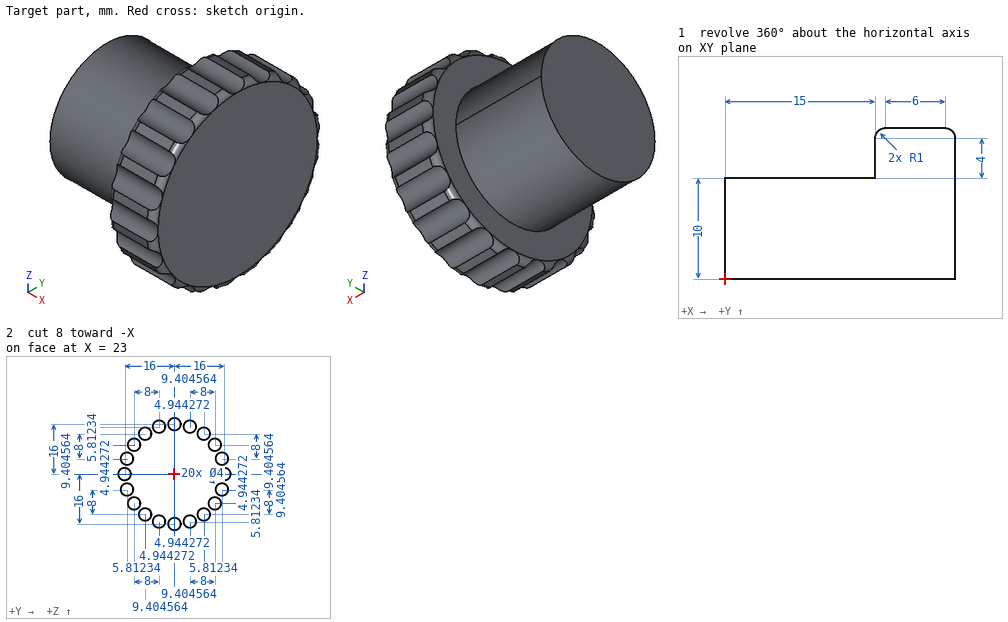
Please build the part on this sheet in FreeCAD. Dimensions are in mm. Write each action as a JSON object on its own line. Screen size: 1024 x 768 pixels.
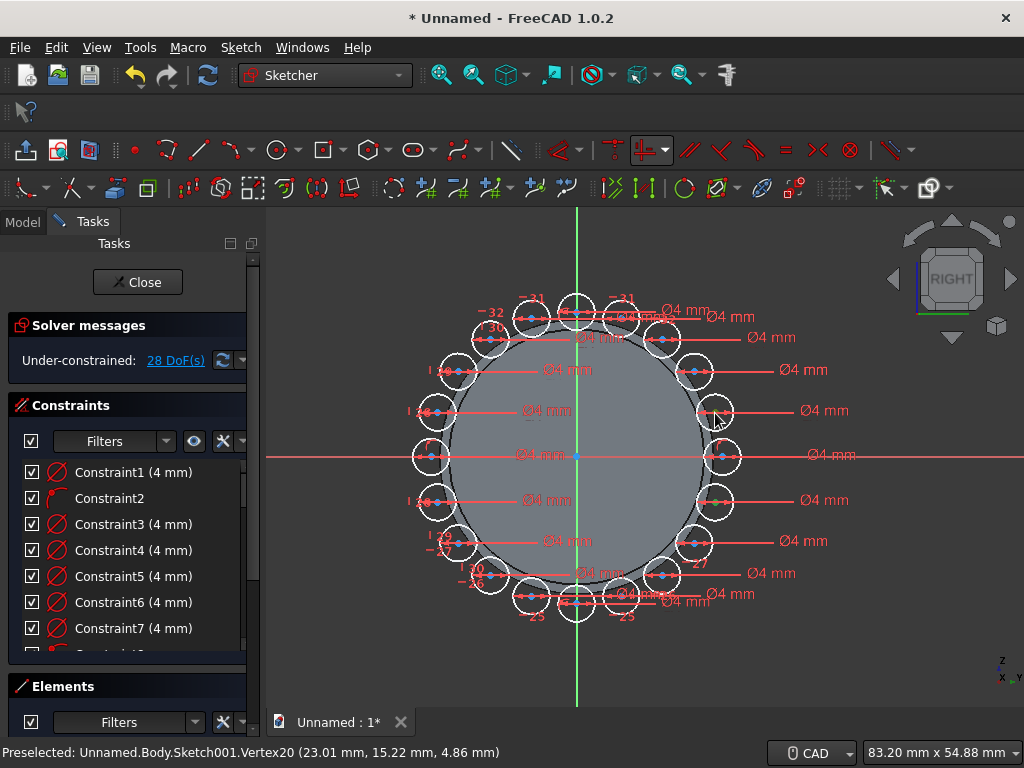
{"action": "left_click", "coordinate": [668, 150]}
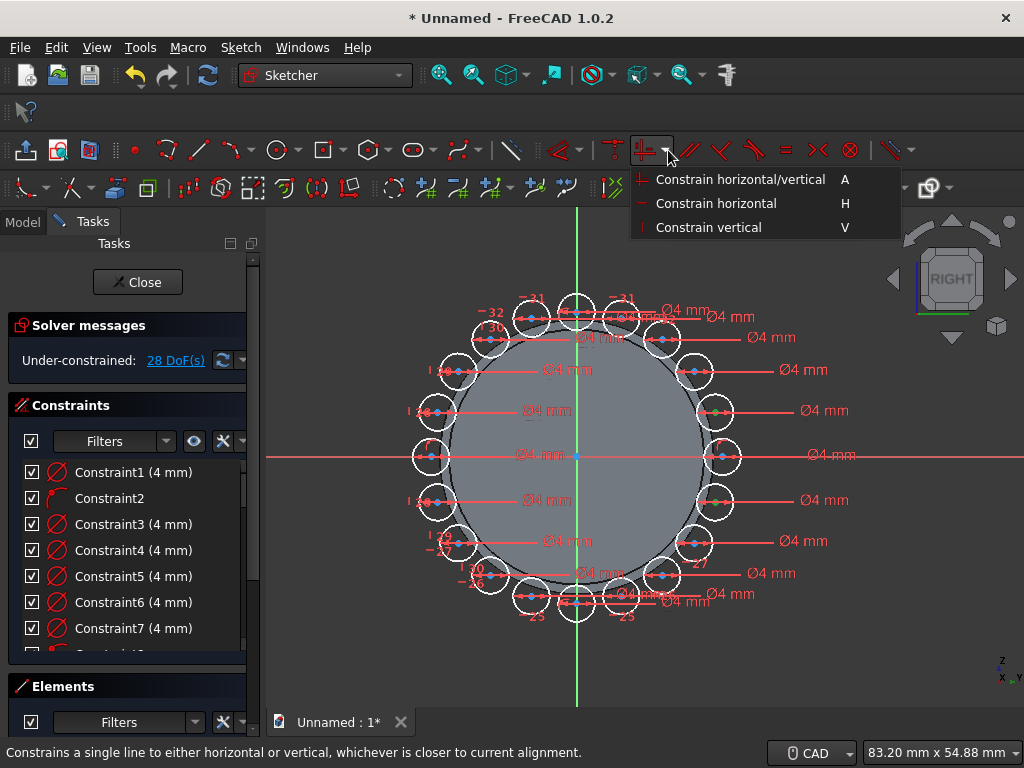
{"action": "left_click", "coordinate": [766, 227]}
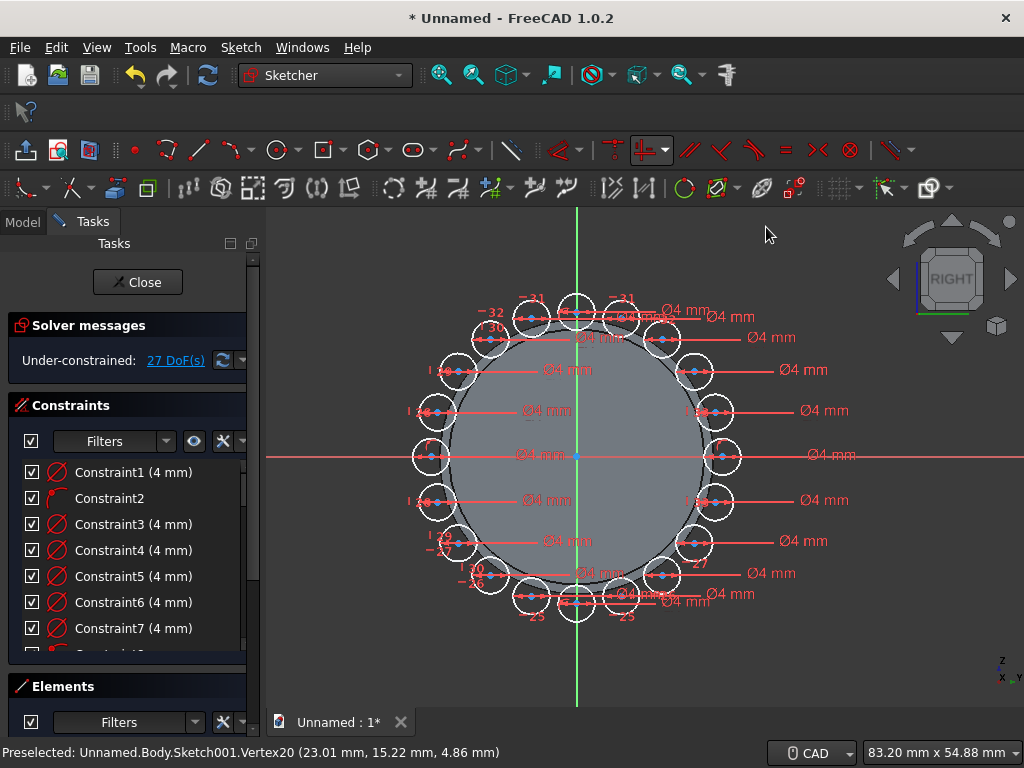
{"action": "left_click", "coordinate": [558, 150]}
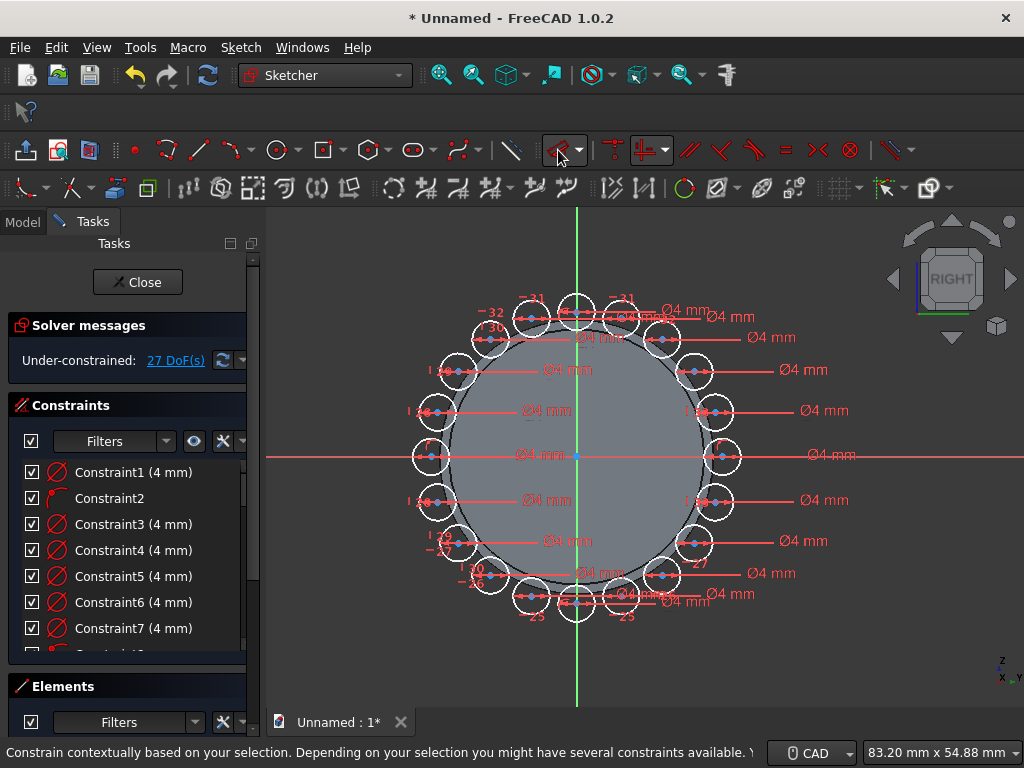
{"action": "left_click", "coordinate": [723, 457]}
{"action": "left_click", "coordinate": [650, 491]}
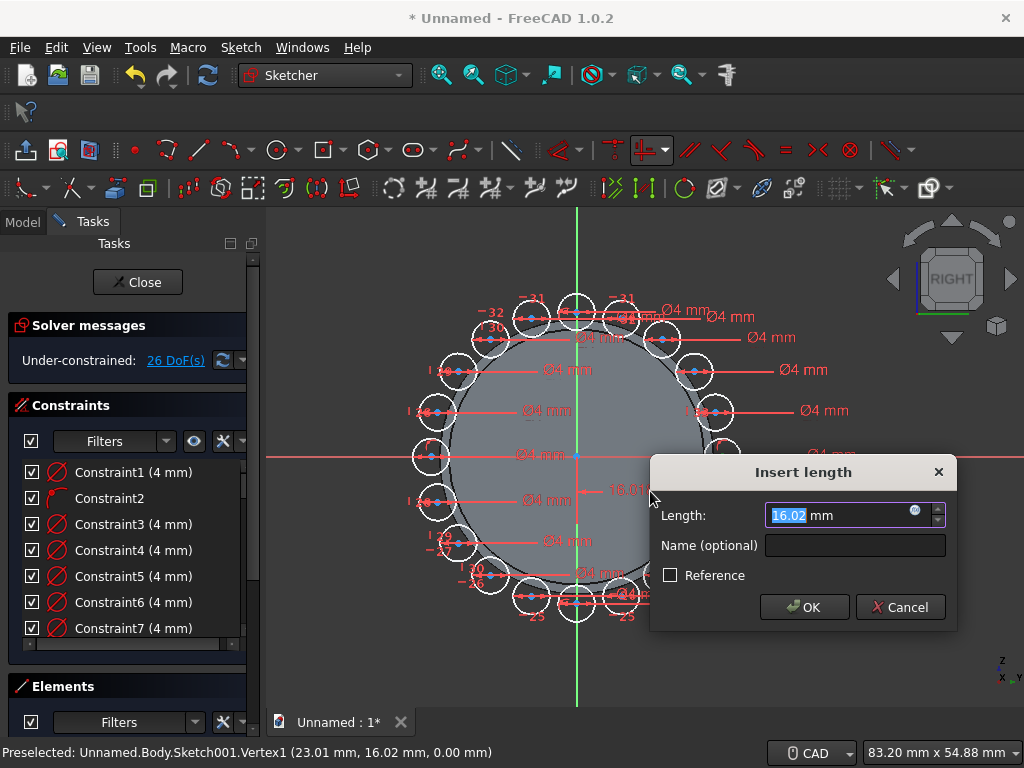
{"action": "type", "text": "16"}
{"action": "key", "text": "Return"}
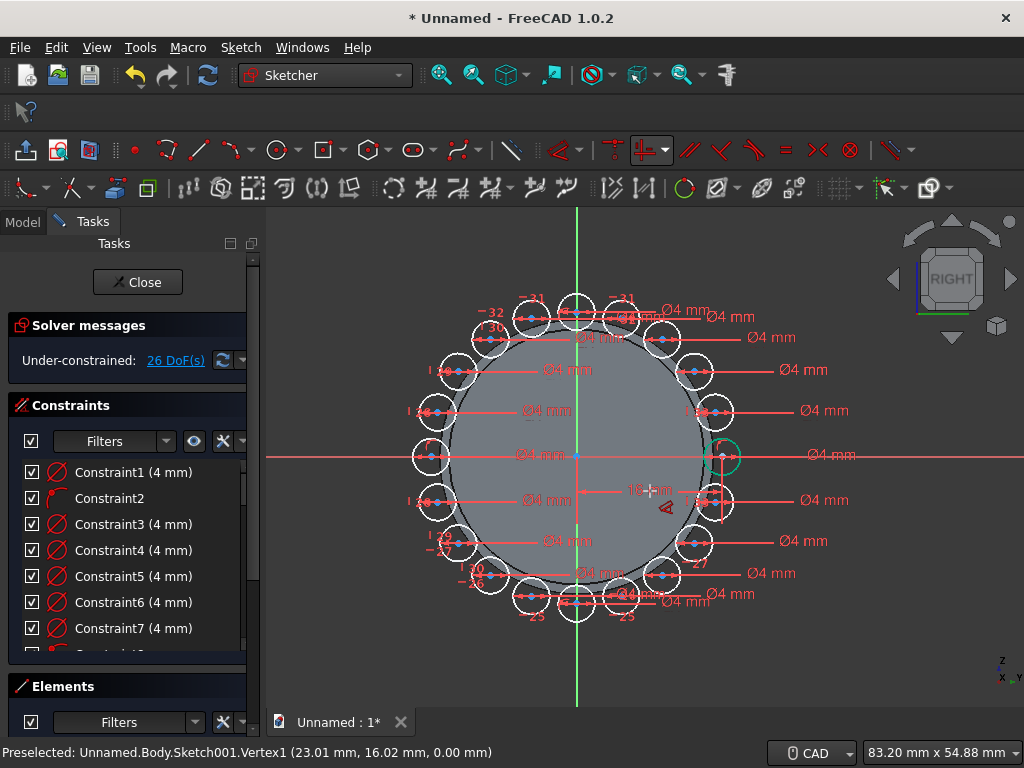
{"action": "left_click", "coordinate": [577, 604]}
{"action": "left_click", "coordinate": [611, 530]}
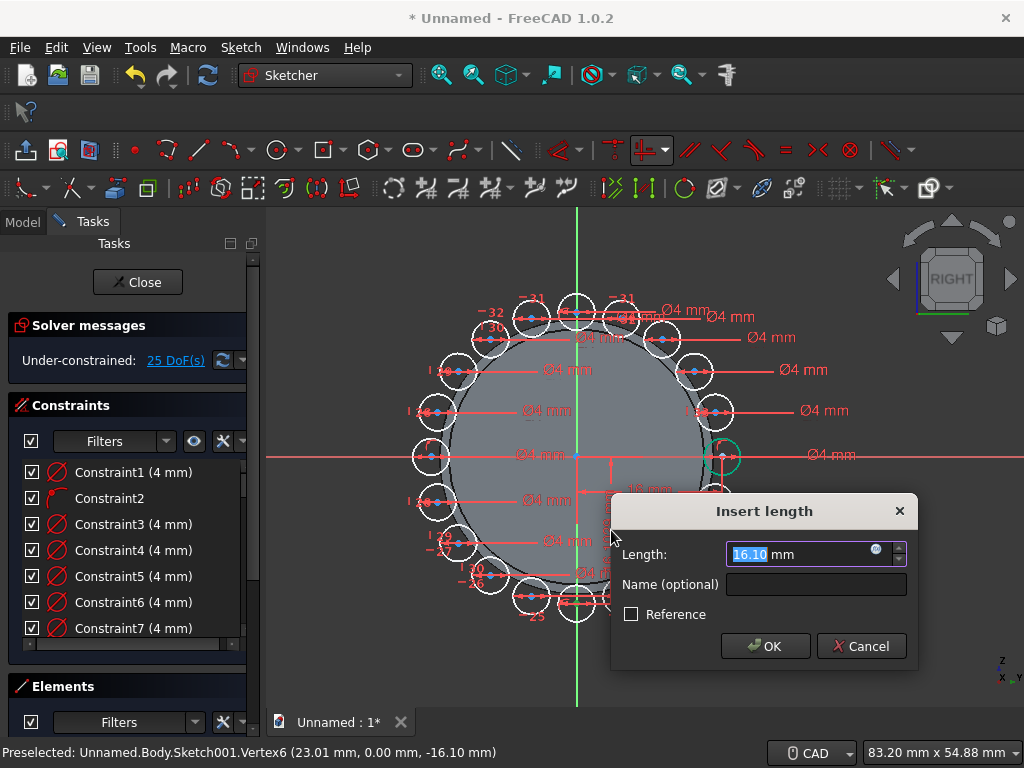
{"action": "type", "text": "16"}
{"action": "key", "text": "Return"}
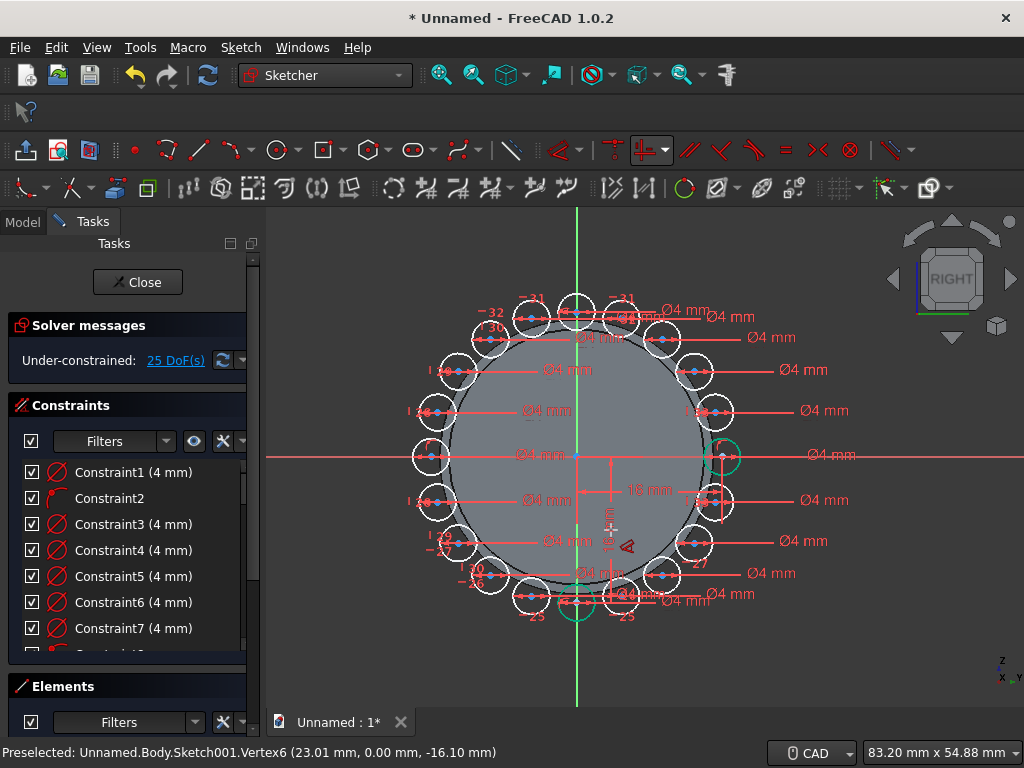
{"action": "left_click", "coordinate": [431, 457]}
{"action": "left_click", "coordinate": [504, 491]}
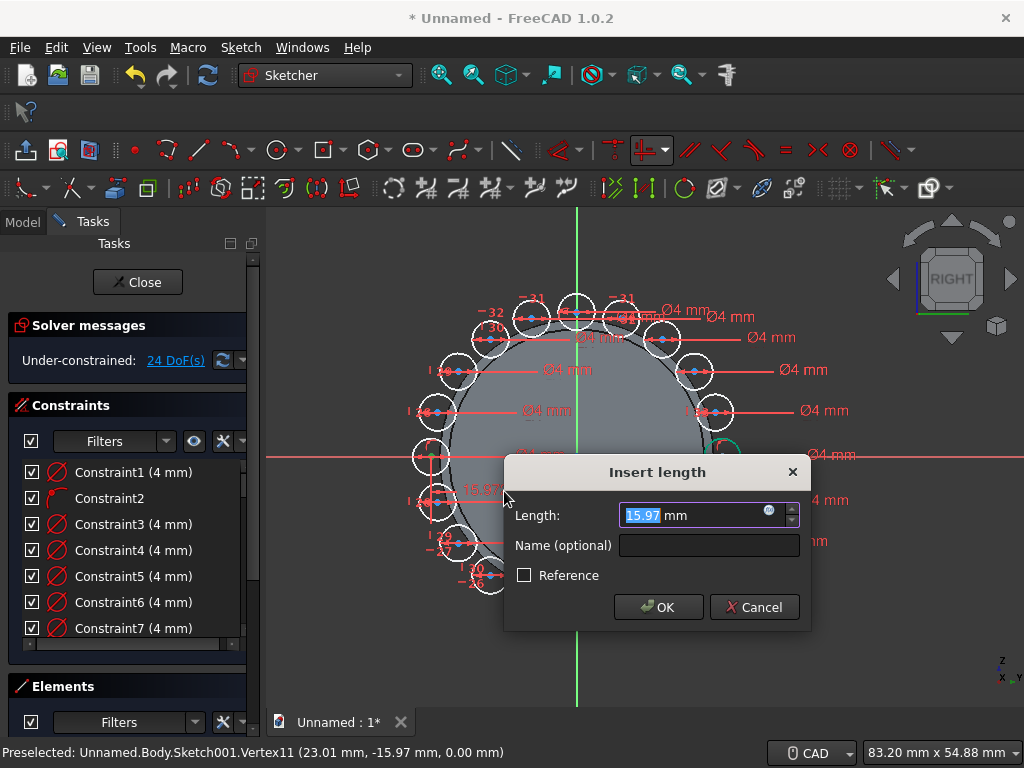
{"action": "type", "text": "16"}
{"action": "key", "text": "Return"}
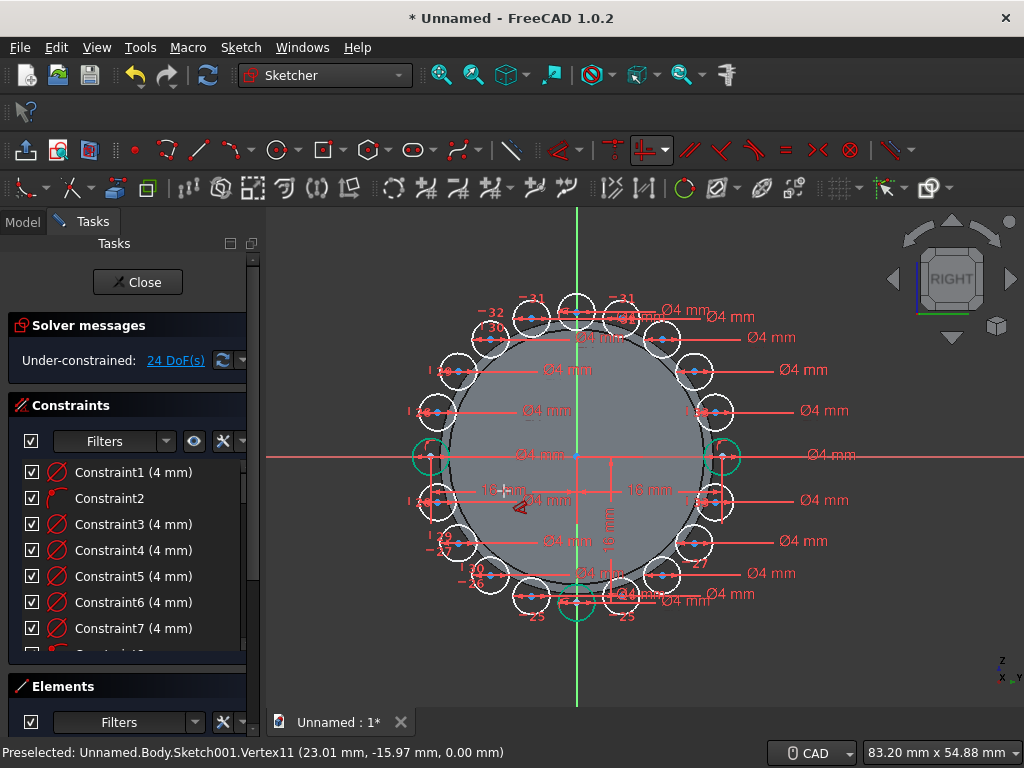
{"action": "left_click", "coordinate": [577, 312]}
{"action": "left_click", "coordinate": [611, 384]}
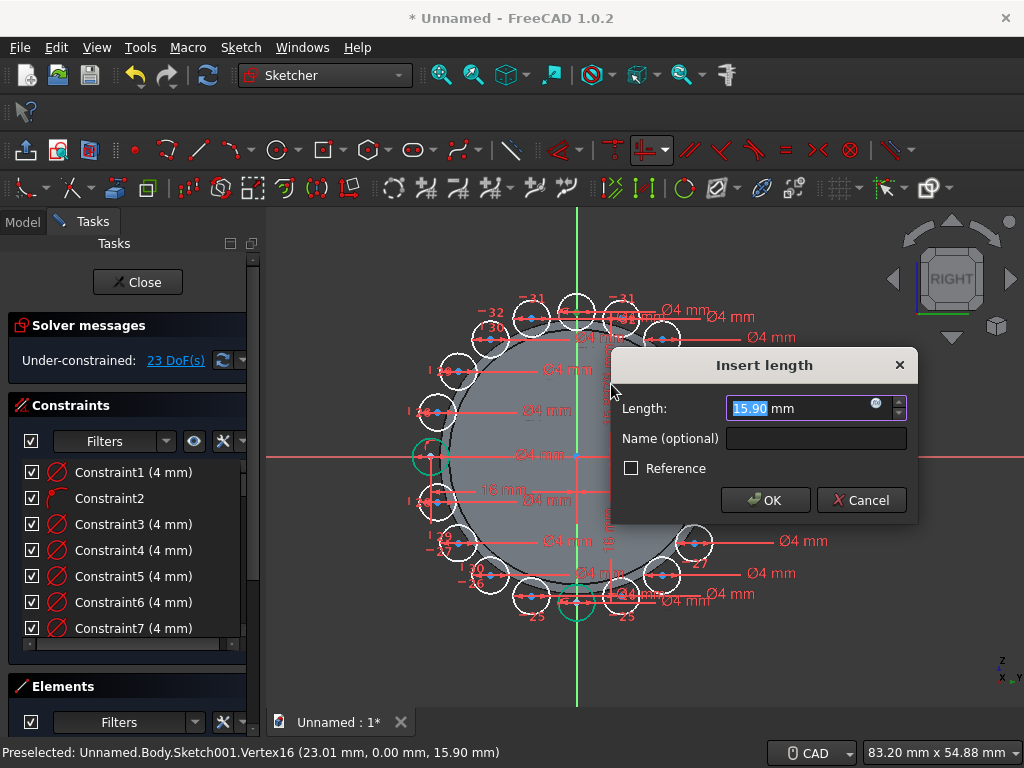
{"action": "type", "text": "16"}
{"action": "key", "text": "Return"}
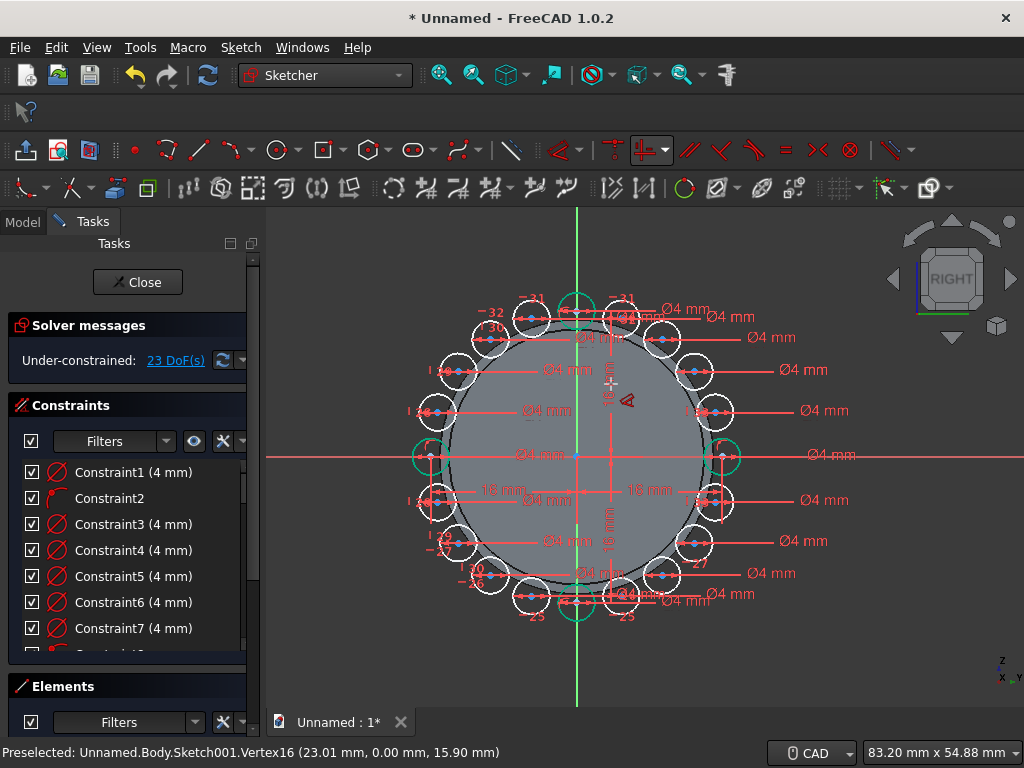
{"action": "left_click", "coordinate": [715, 502]}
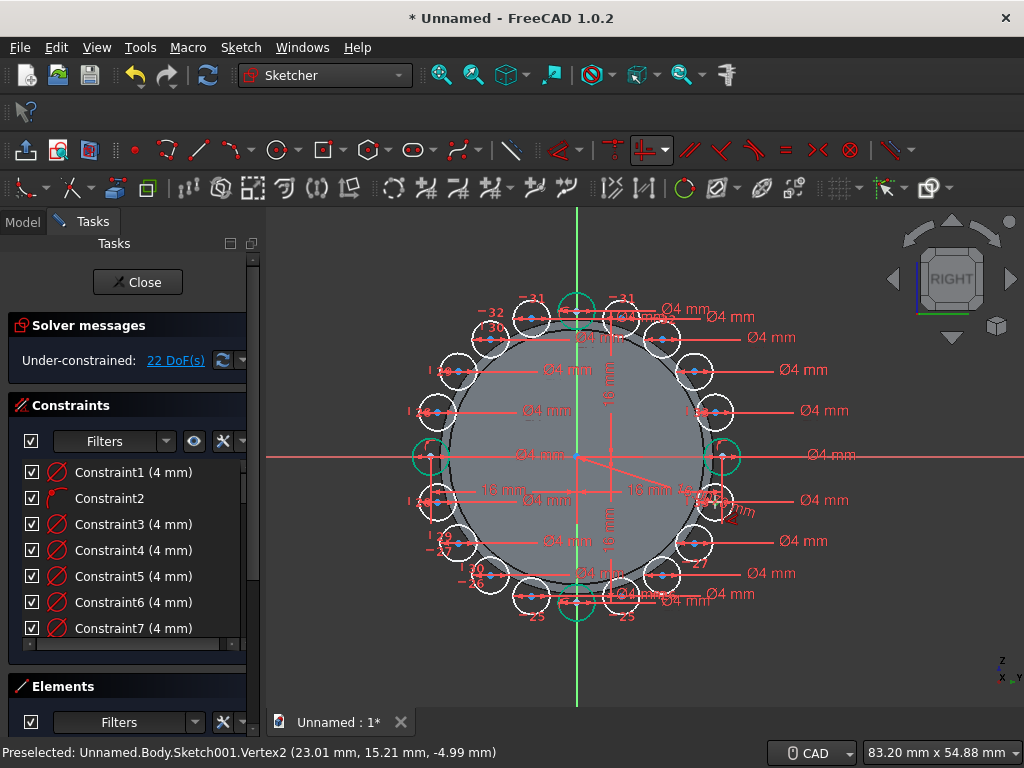
{"action": "left_click", "coordinate": [662, 575]}
{"action": "left_click", "coordinate": [749, 539]}